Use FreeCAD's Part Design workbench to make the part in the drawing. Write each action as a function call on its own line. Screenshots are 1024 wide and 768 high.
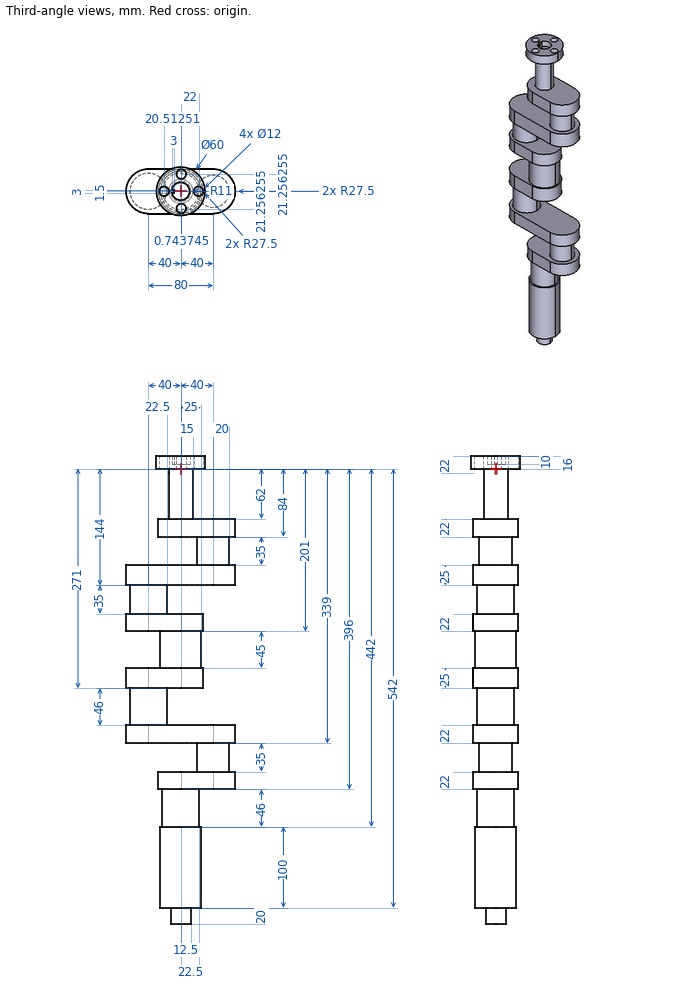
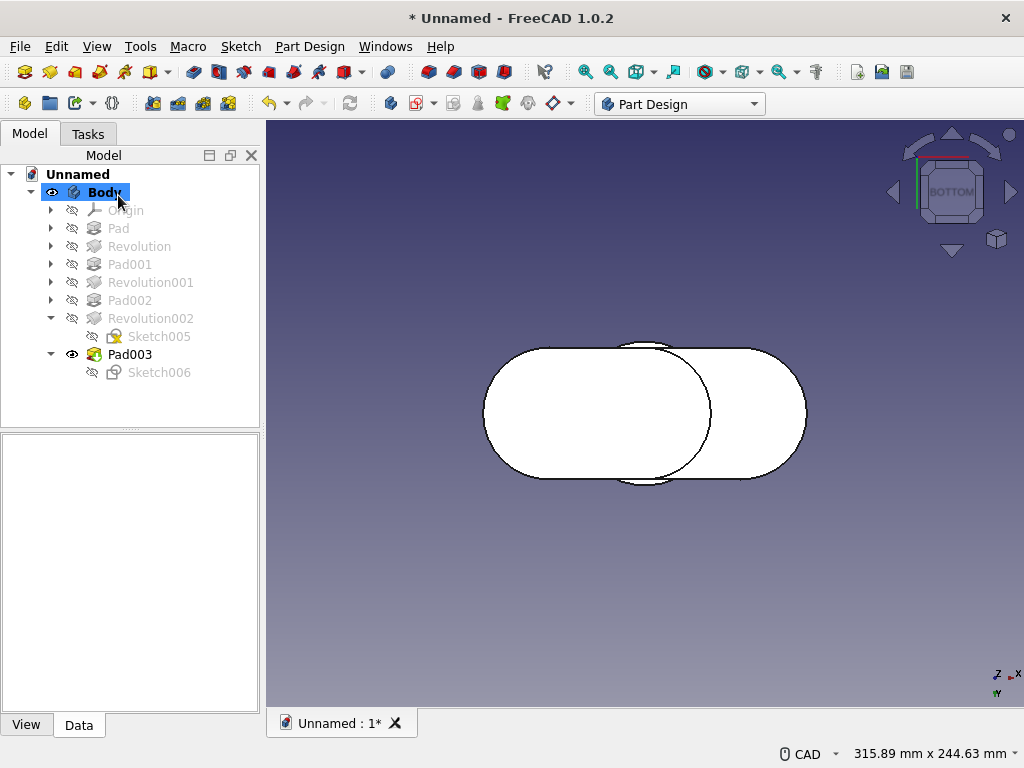
click(586, 72)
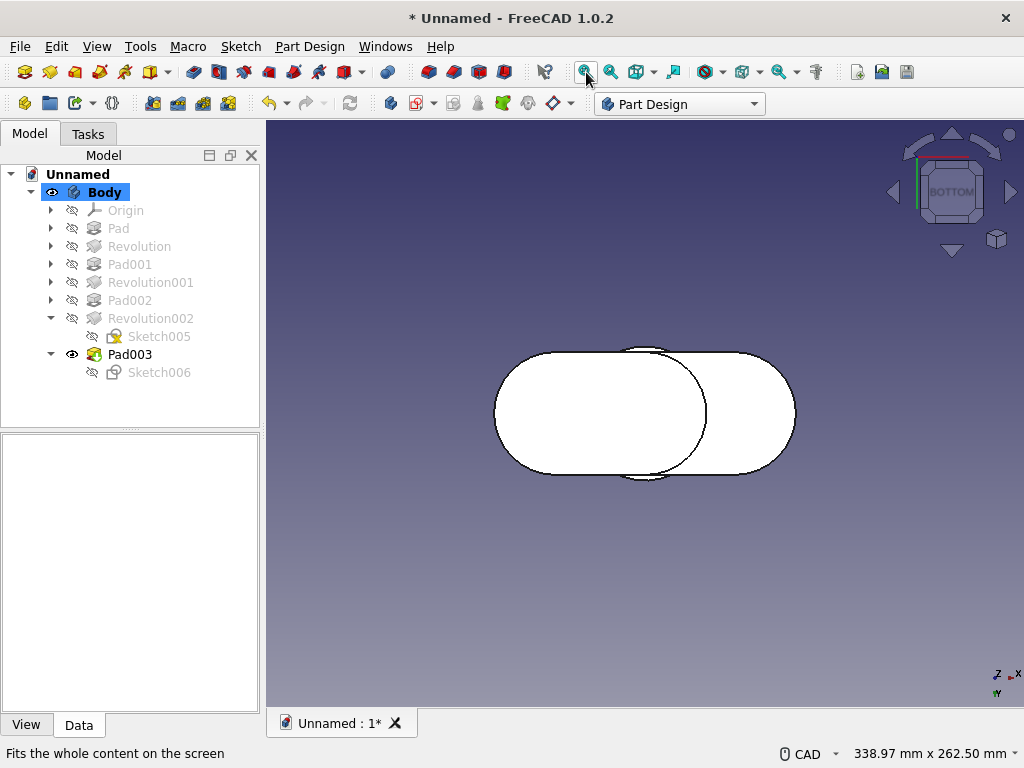
click(416, 104)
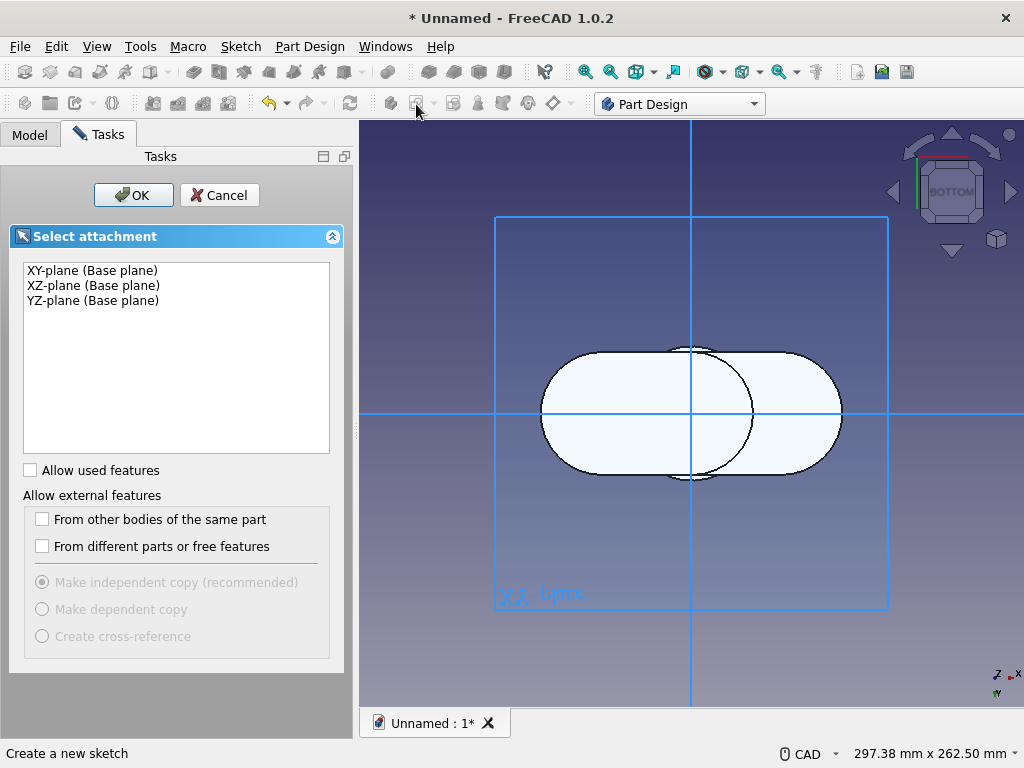
click(84, 286)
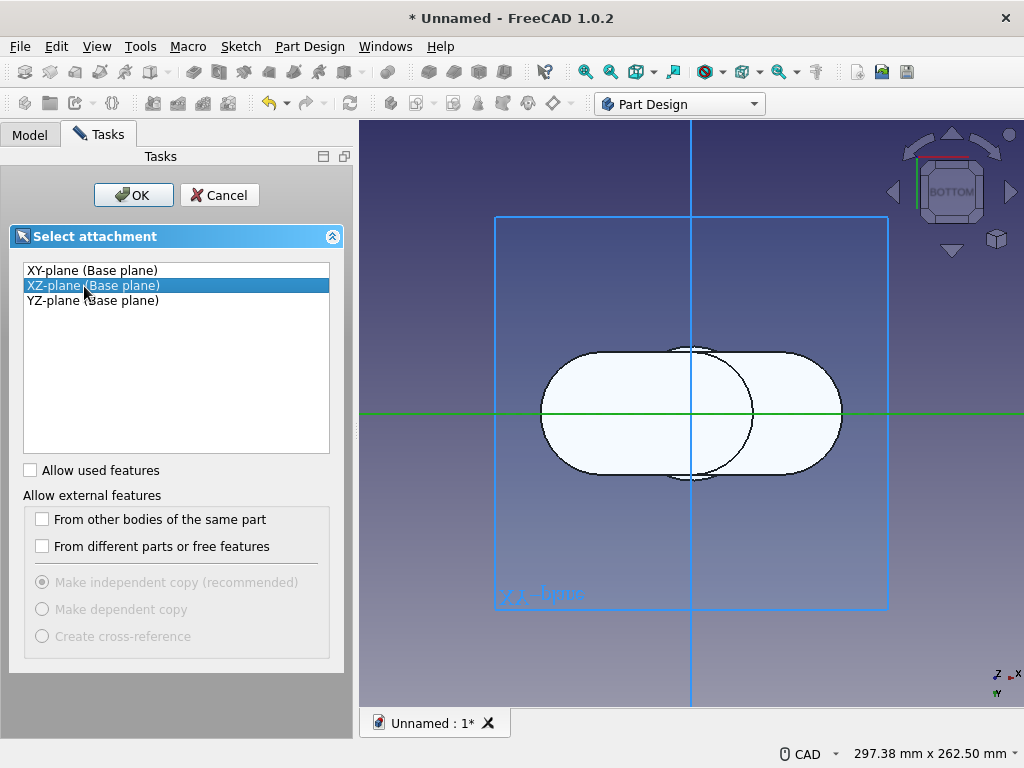
click(134, 195)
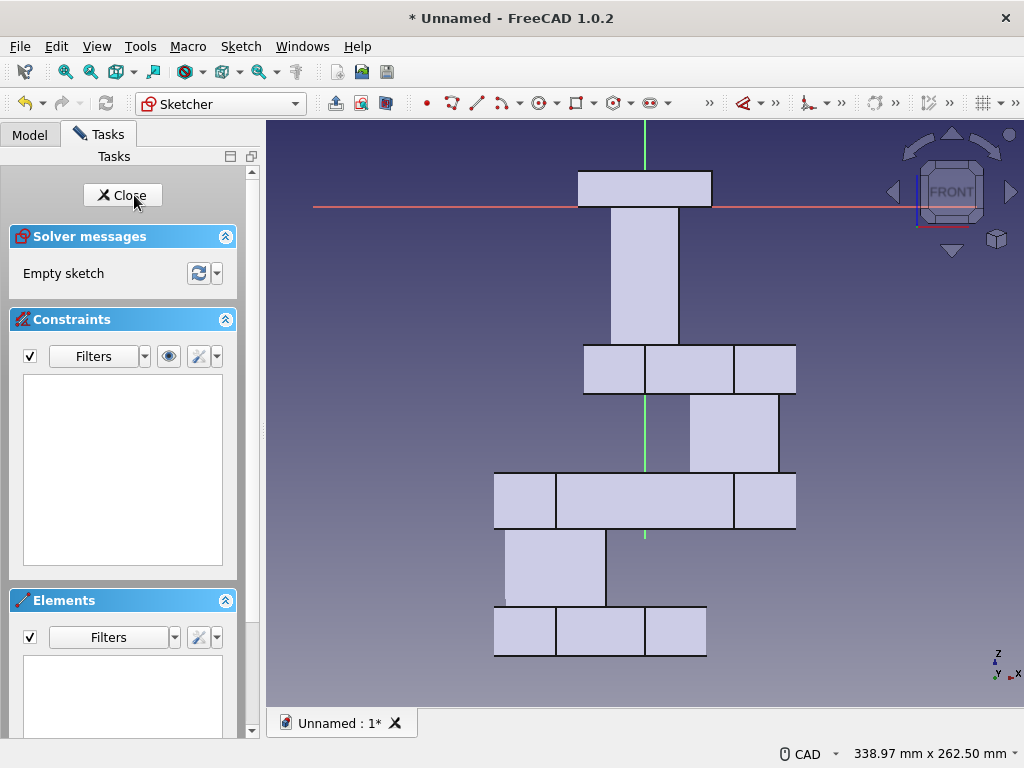
key(q)
key(s)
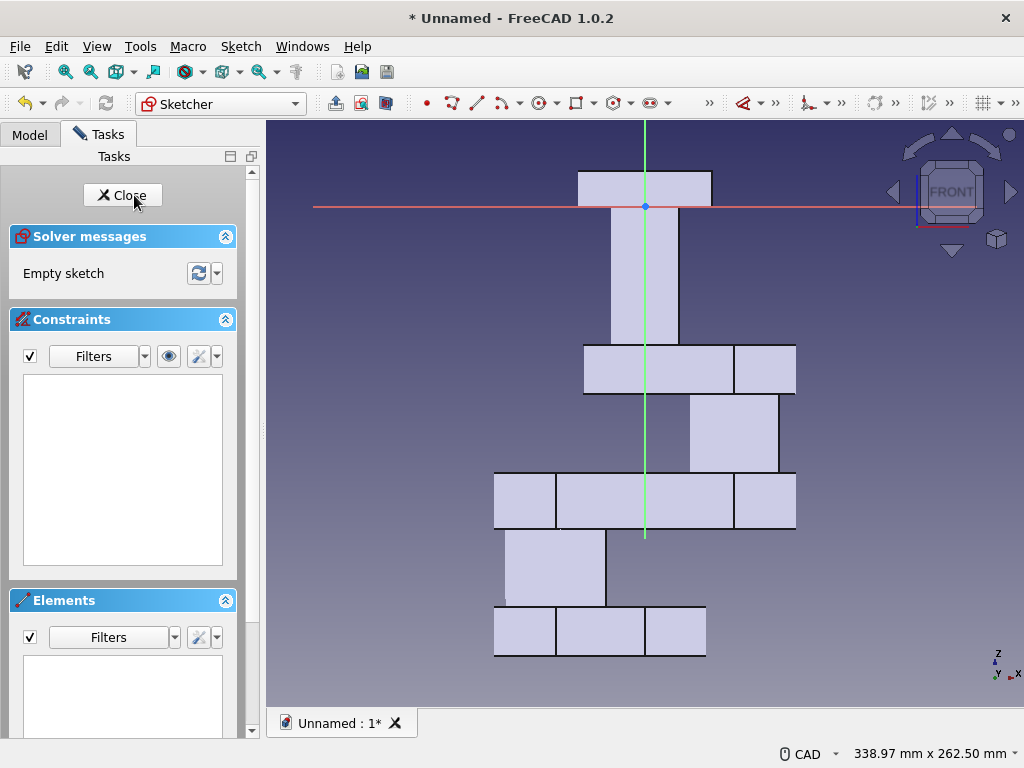
scroll(576, 414, down, 5)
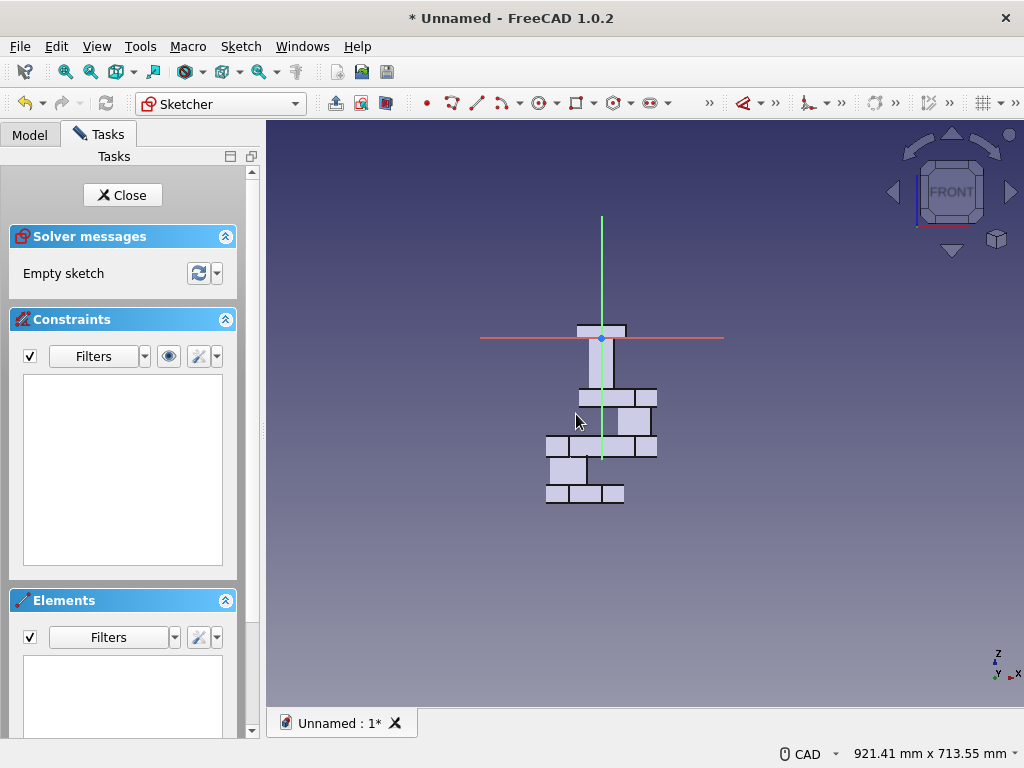
scroll(615, 533, up, 12)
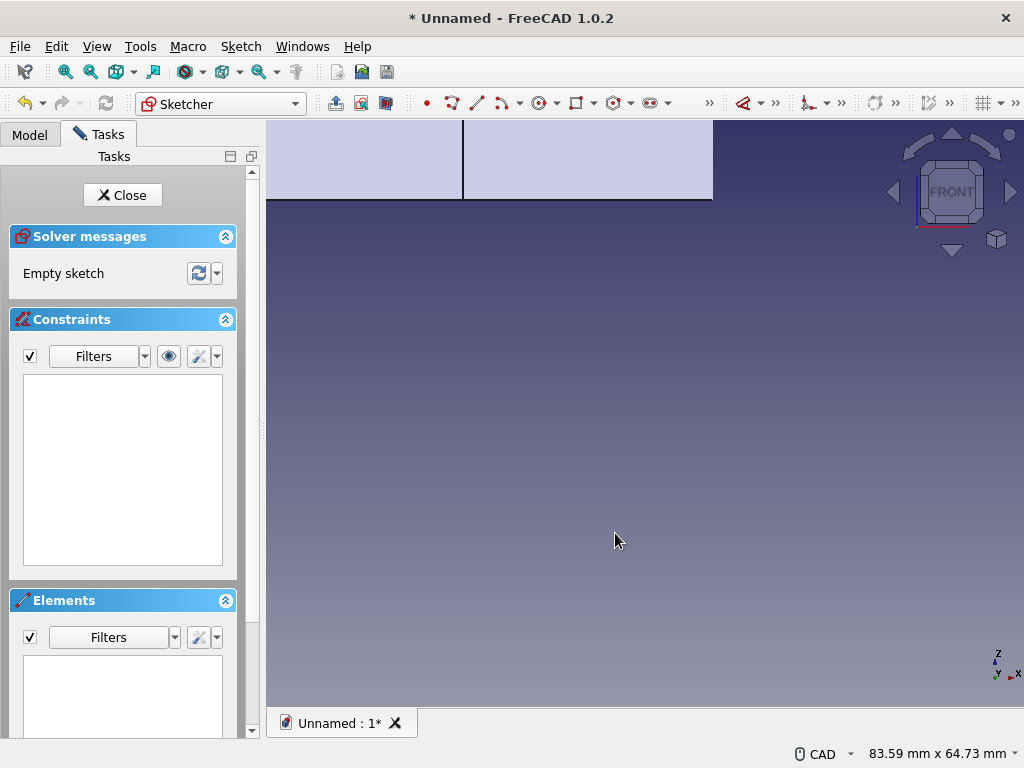
key(g)
key(r)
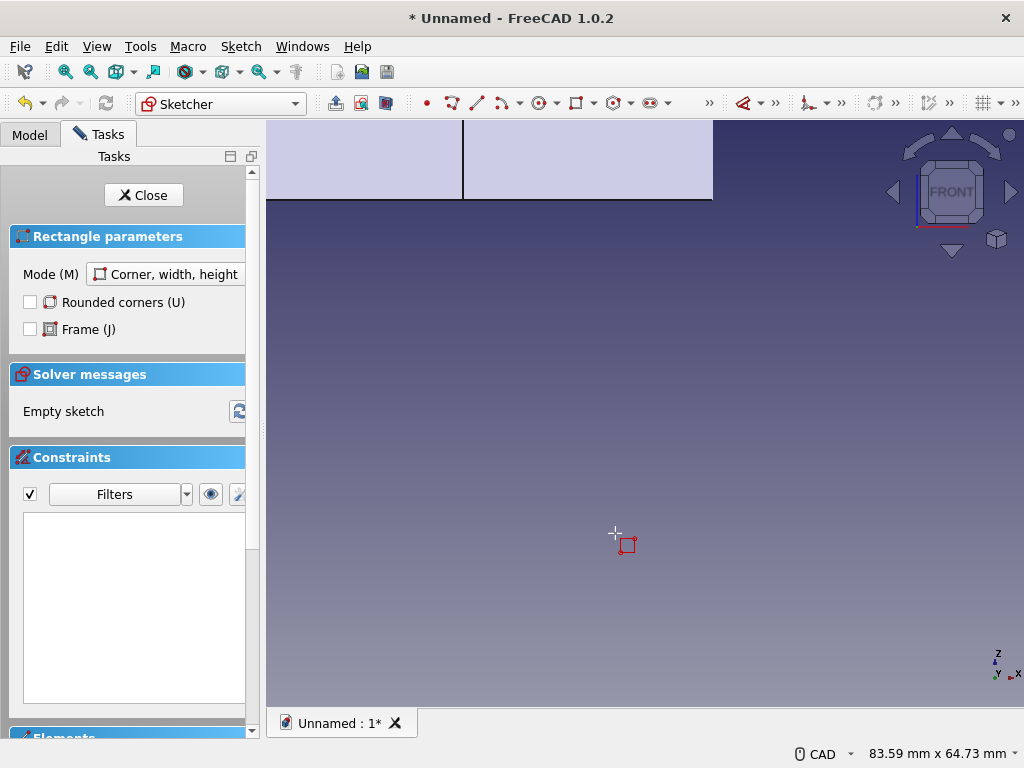
click(463, 200)
move(690, 608)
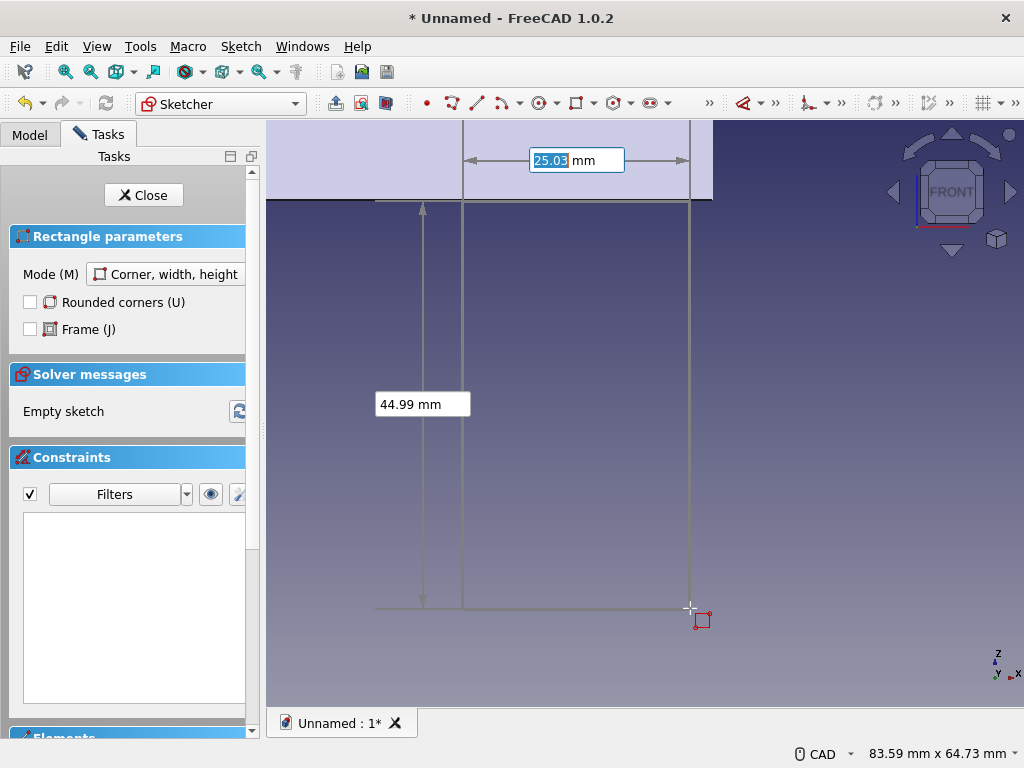
text(25)
key(Tab)
text(45)
key(Return)
key(Escape)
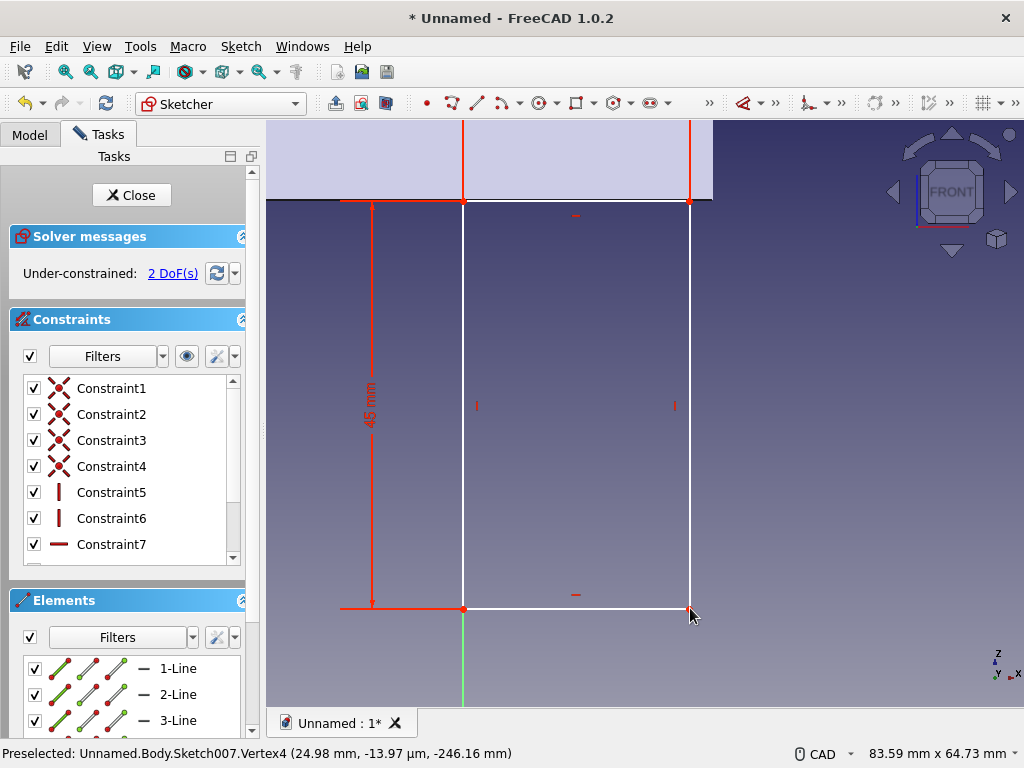
click(463, 201)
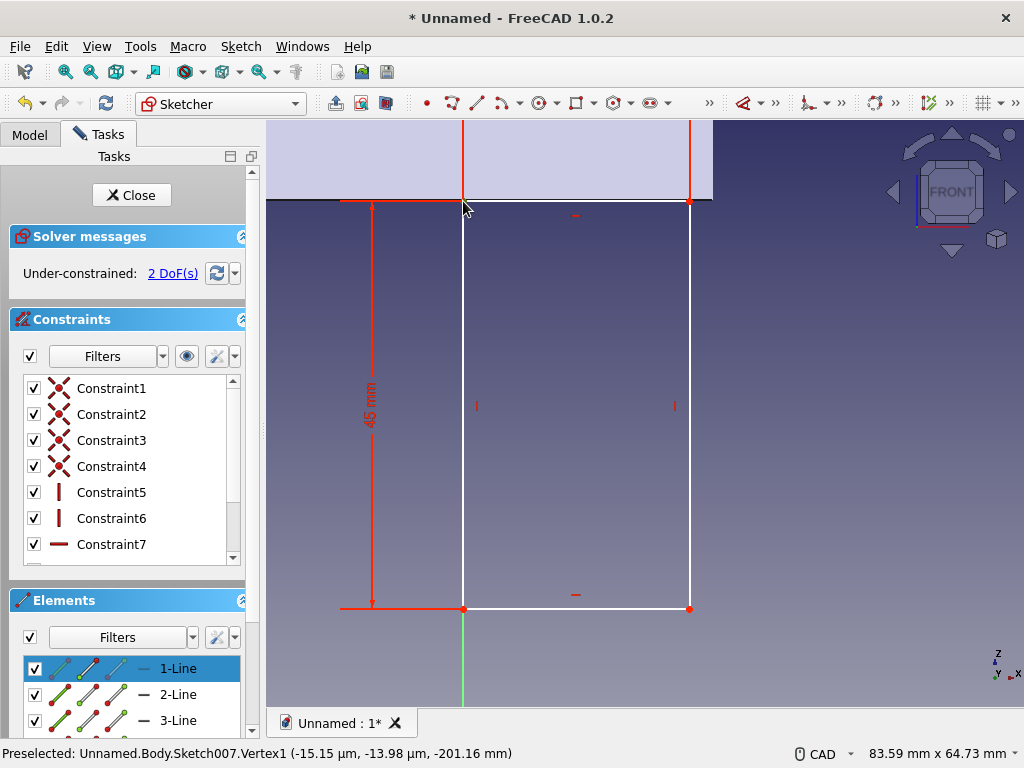
click(463, 641)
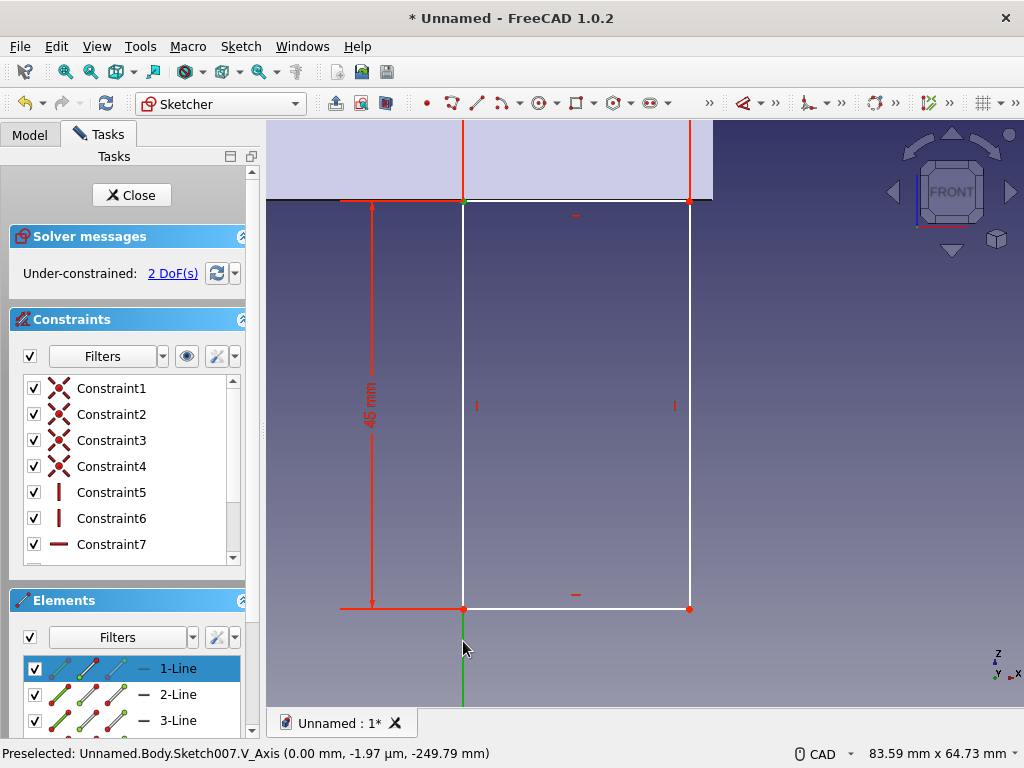
key(c)